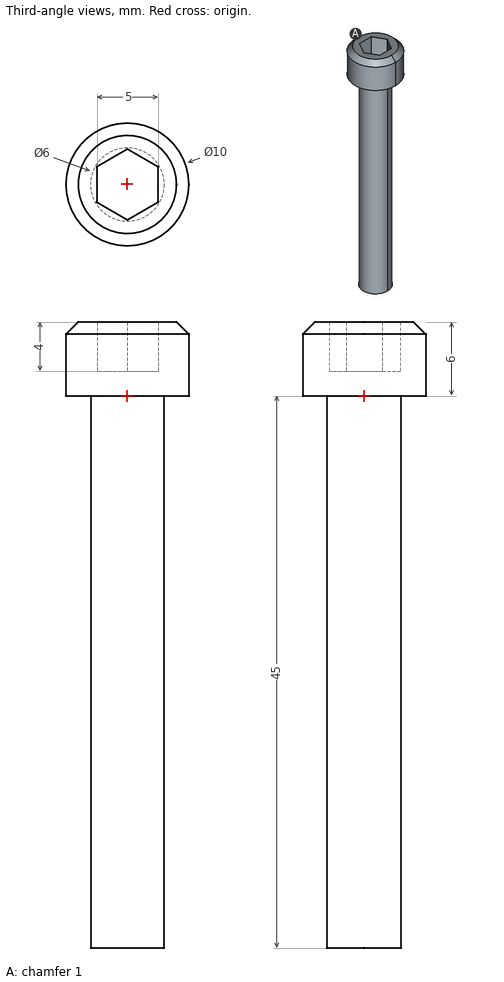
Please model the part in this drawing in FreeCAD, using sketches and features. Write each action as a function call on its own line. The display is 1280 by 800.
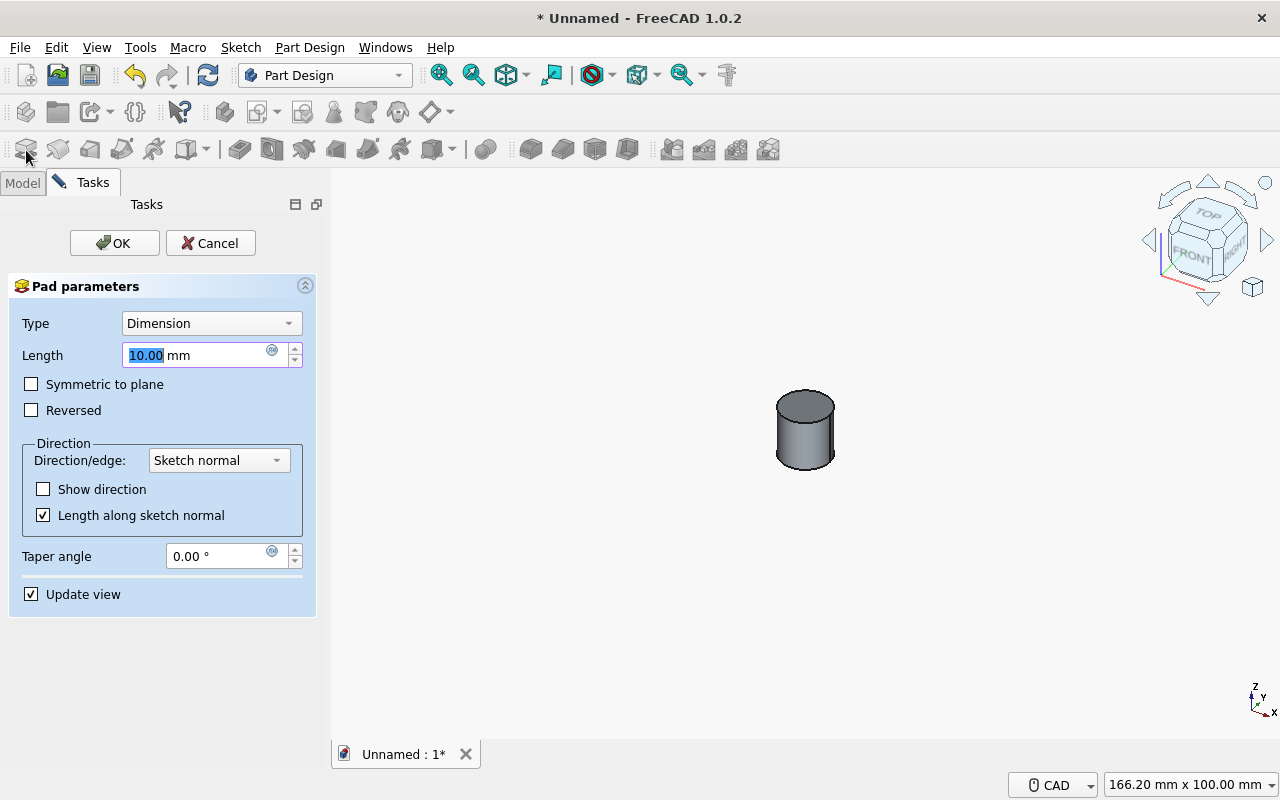
text(6)
key(Tab)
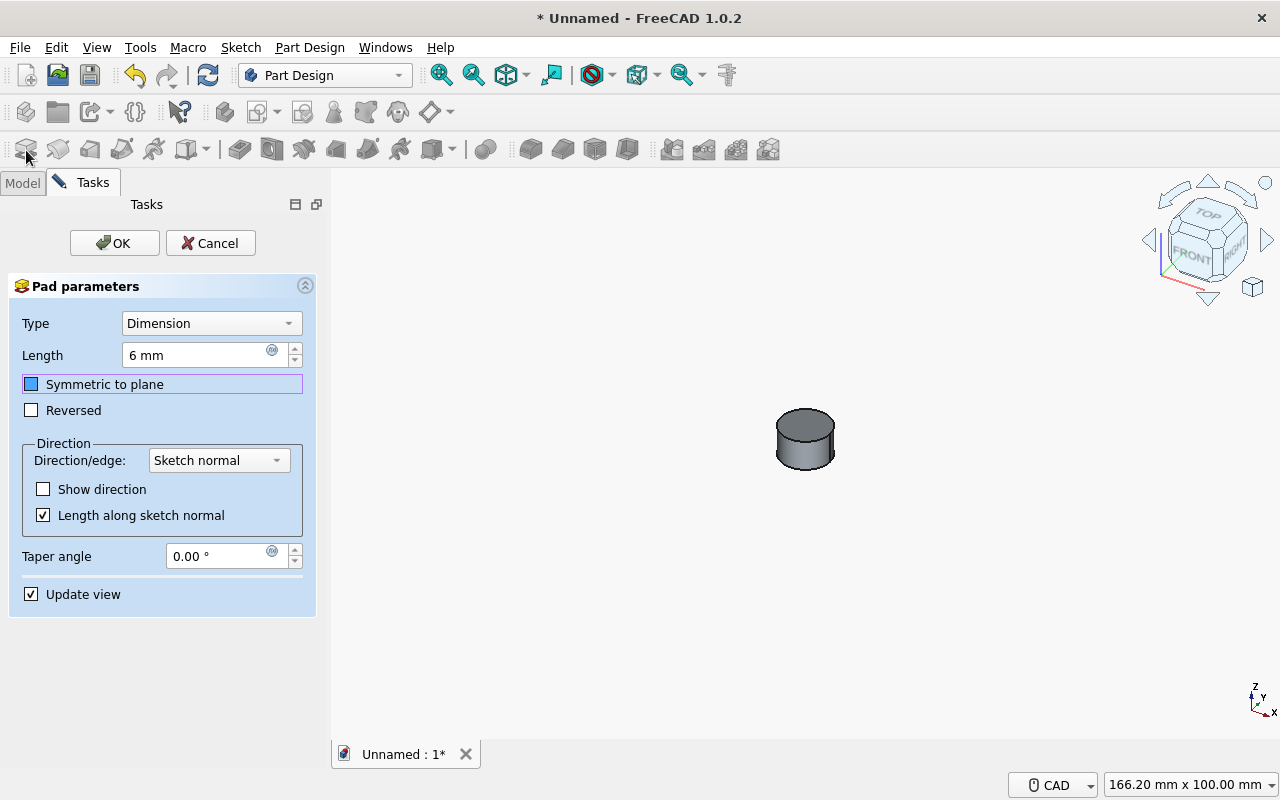
click(115, 243)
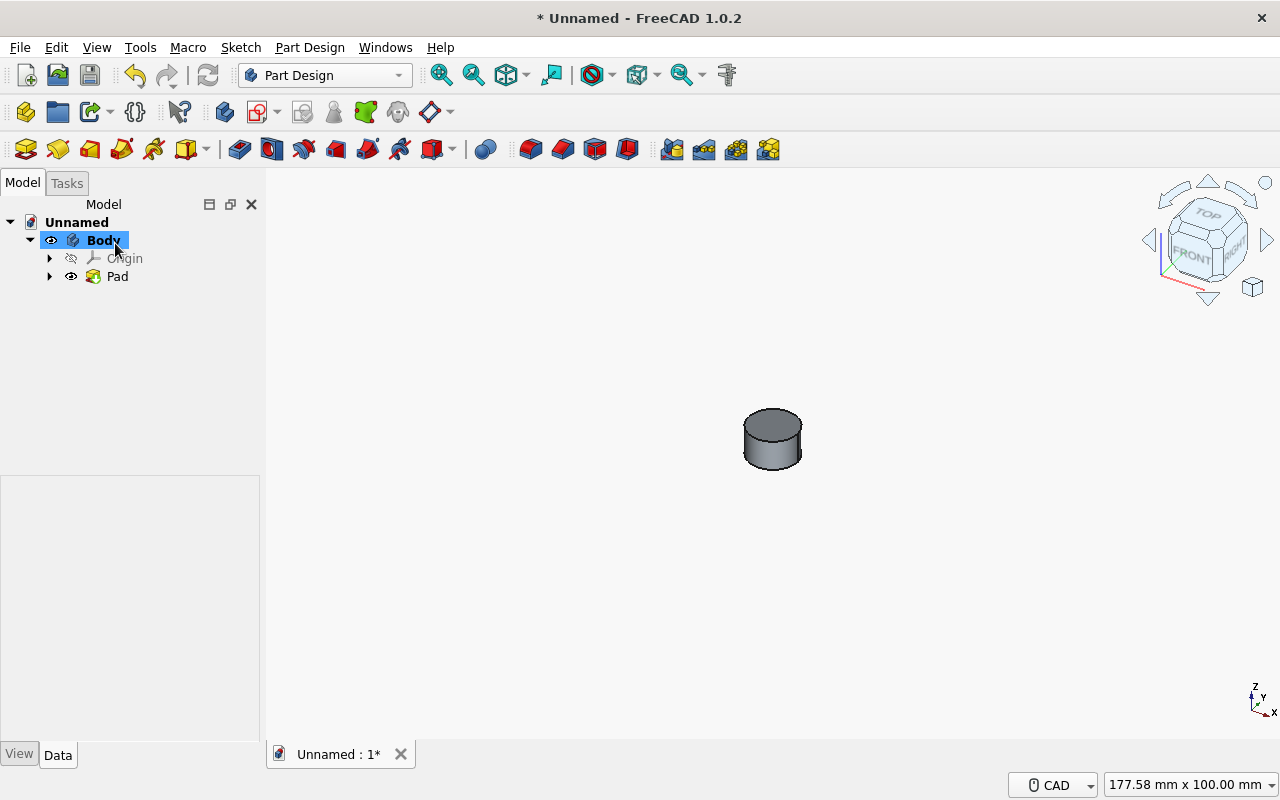
click(442, 76)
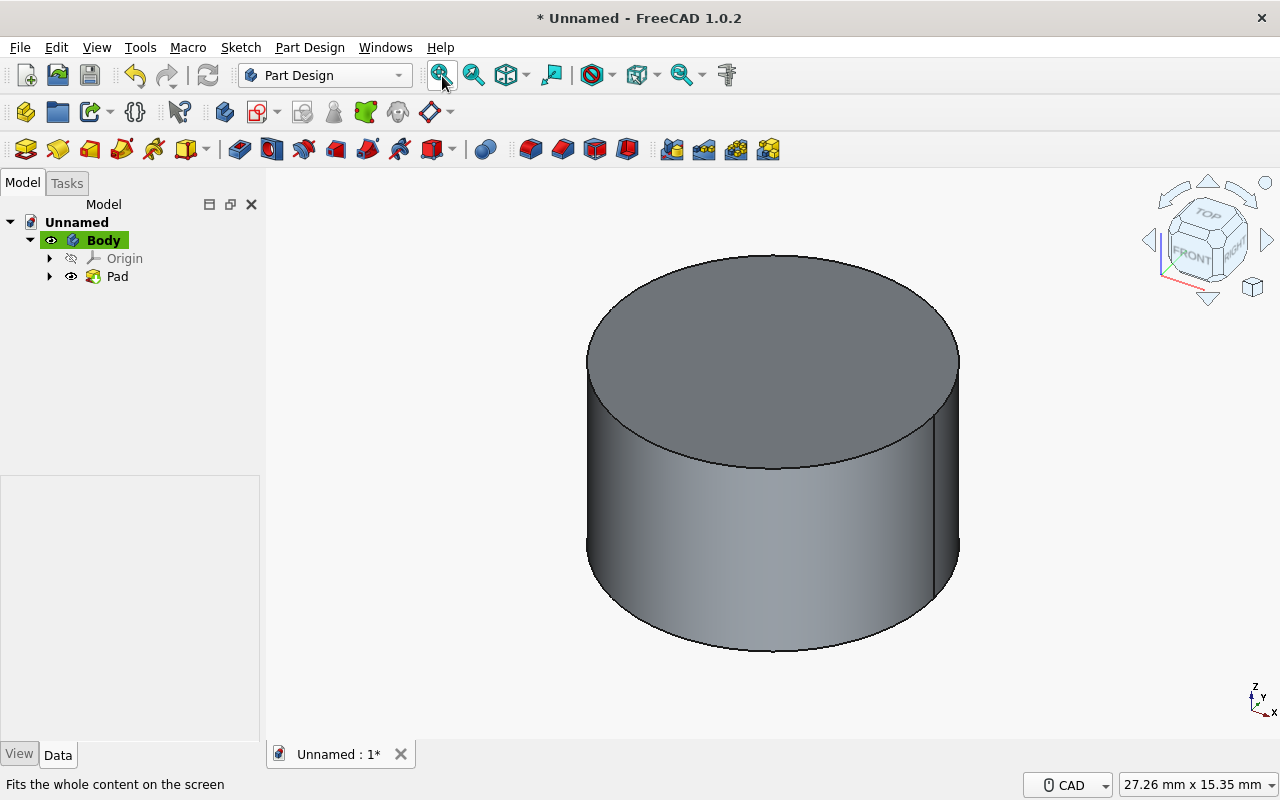
click(773, 361)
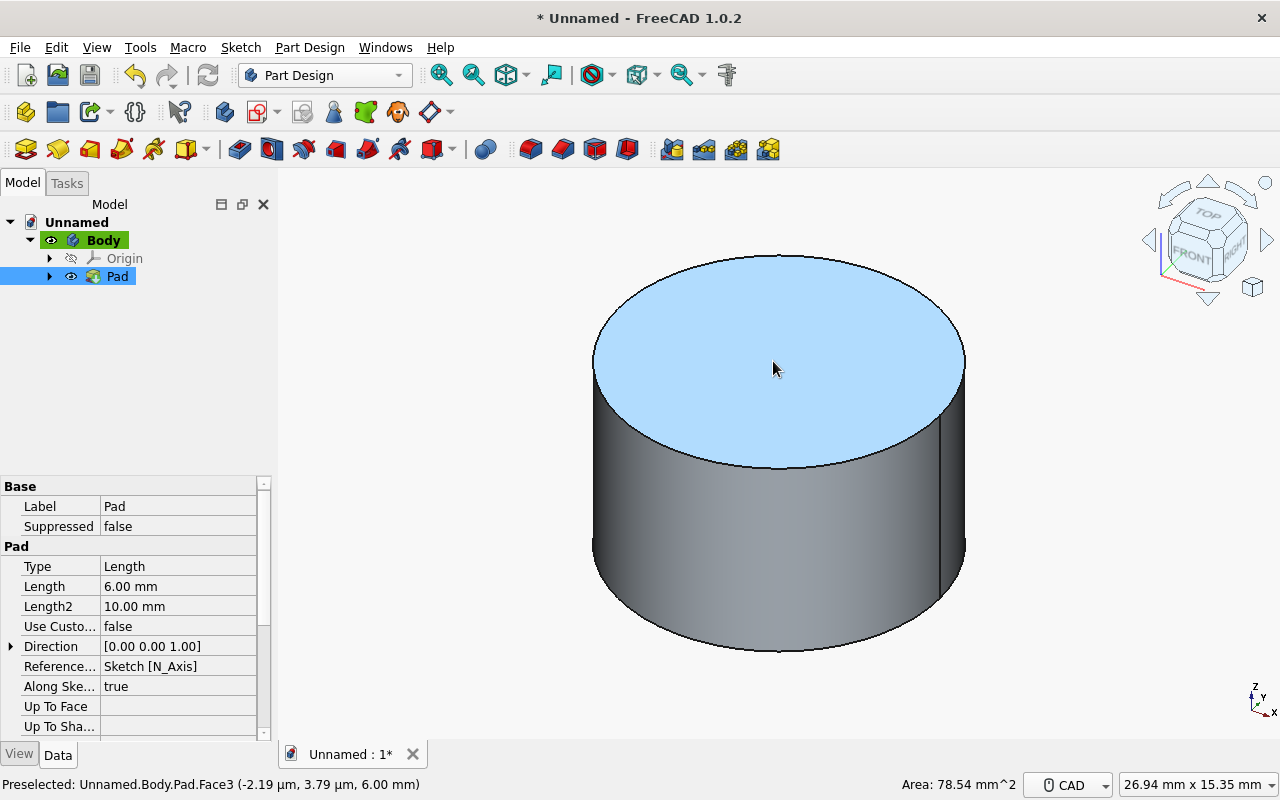
click(258, 112)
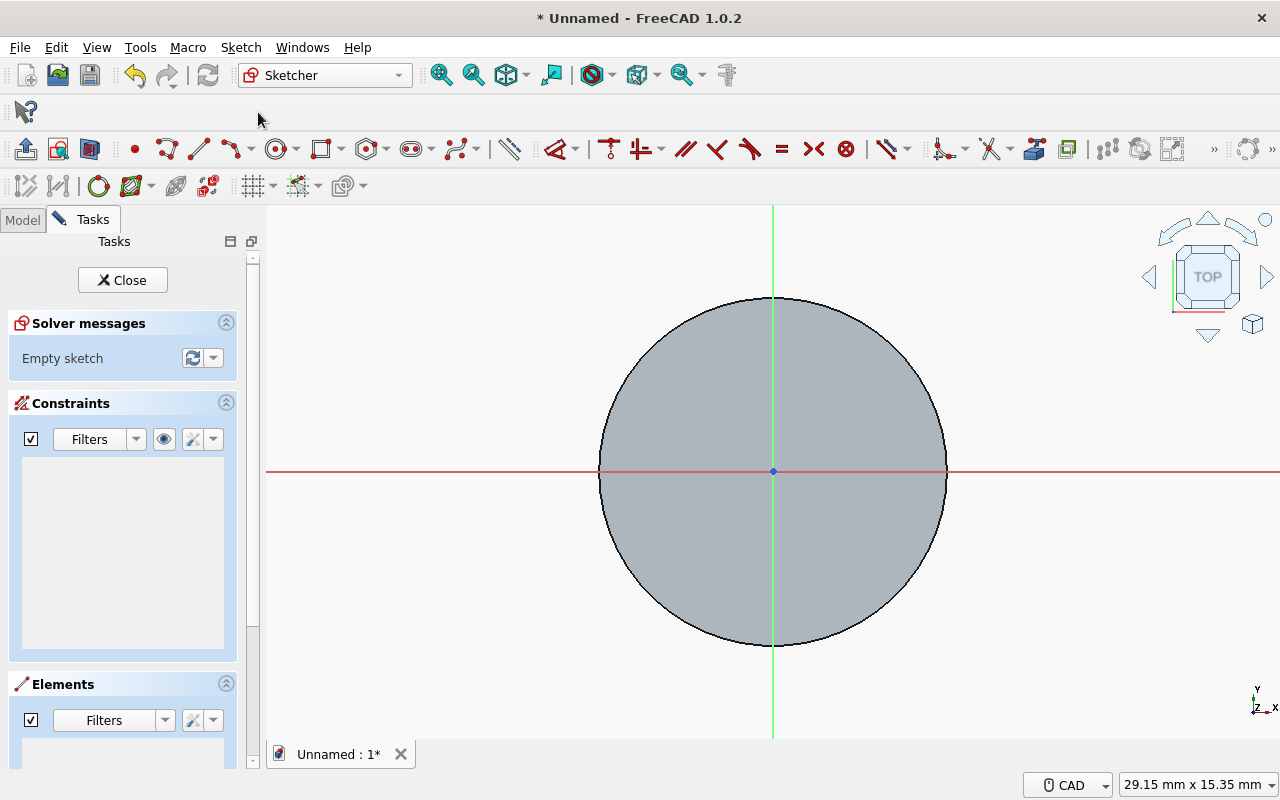
scroll(856, 472, up, 3)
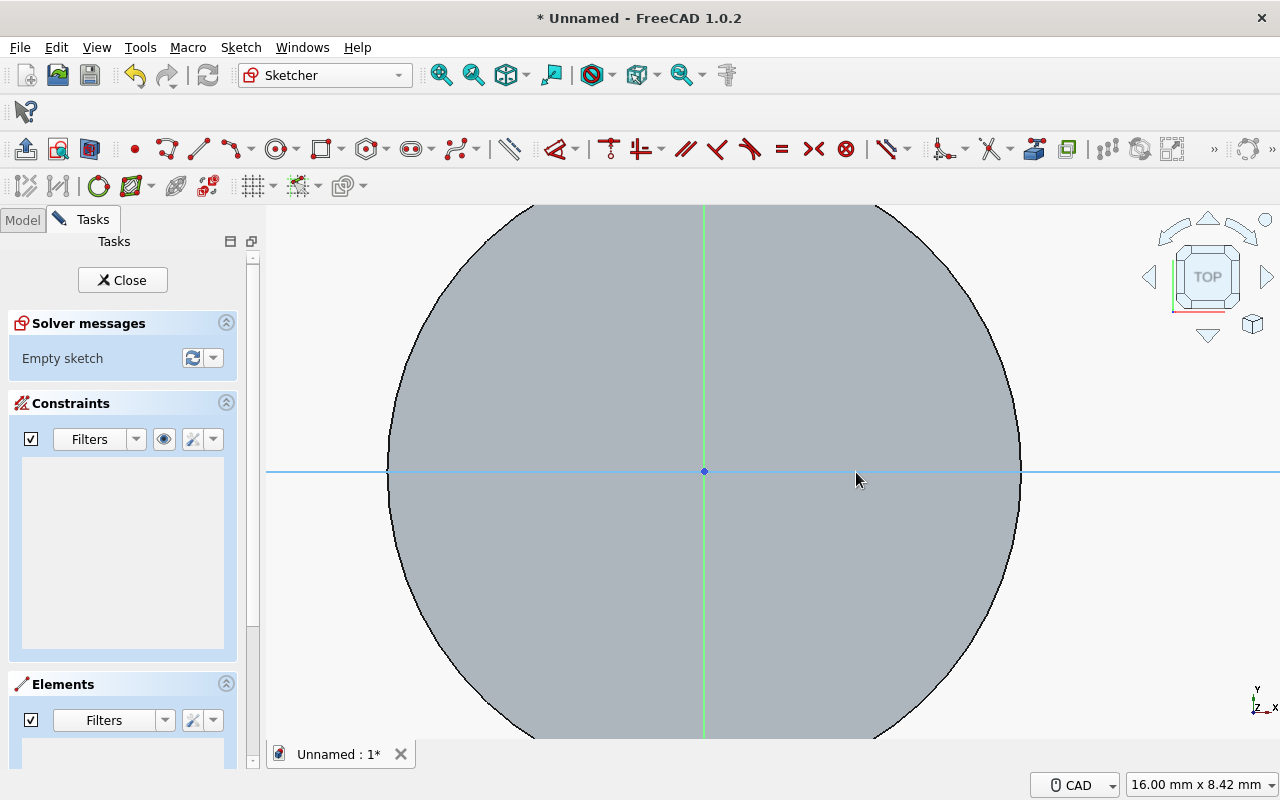
click(366, 150)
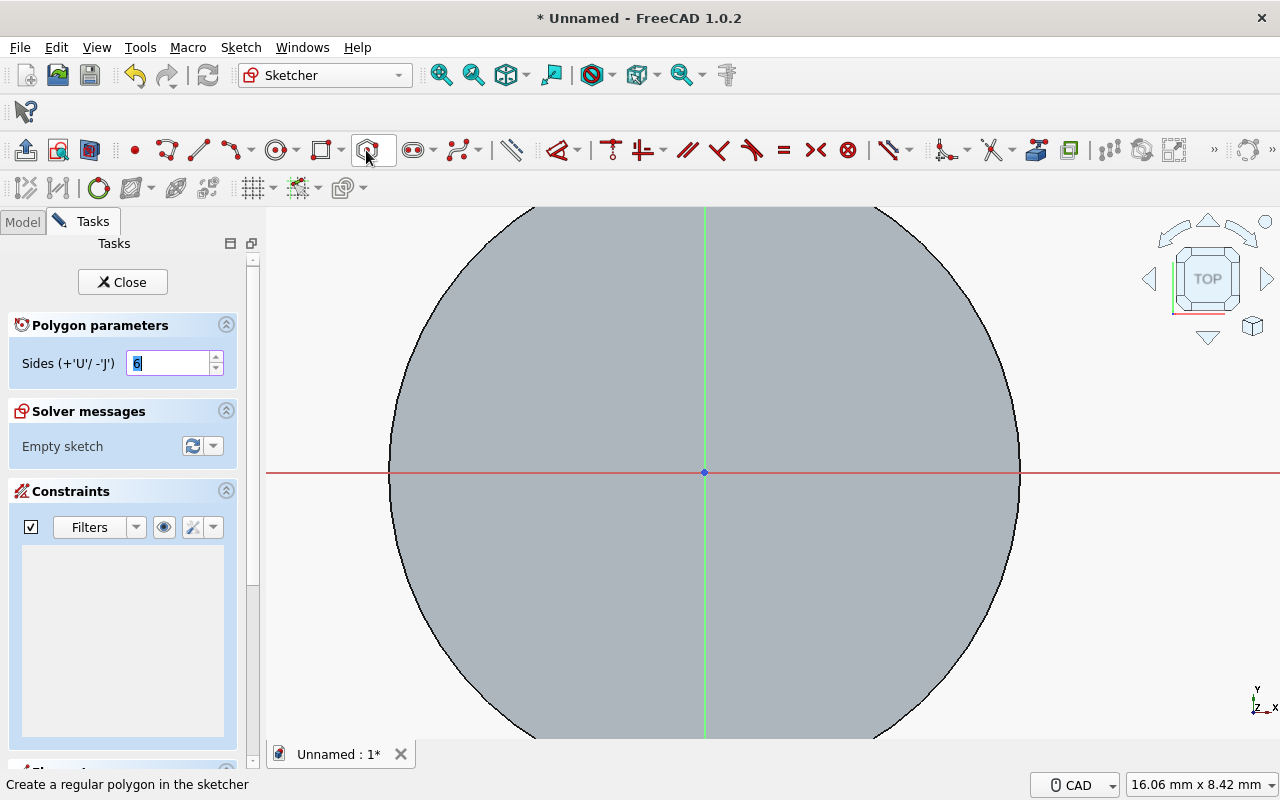
click(705, 473)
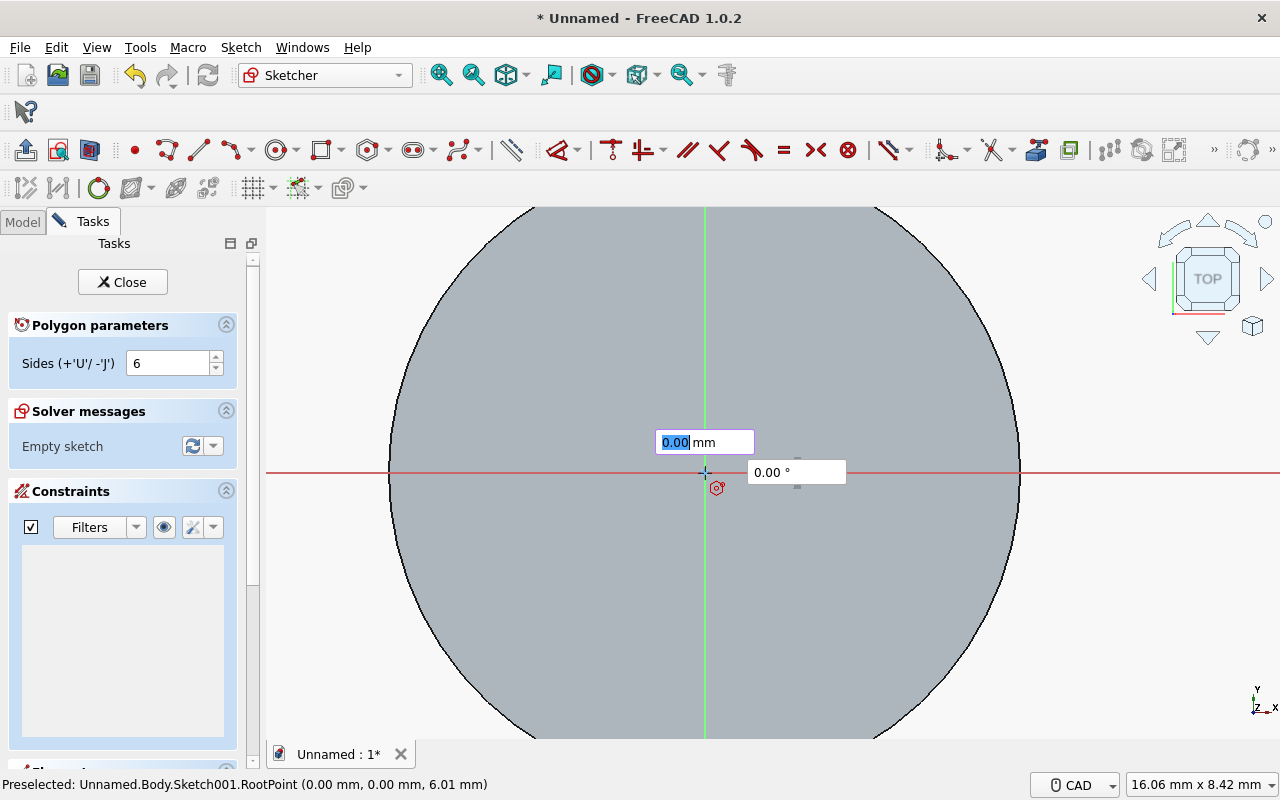
click(705, 290)
right_click(705, 290)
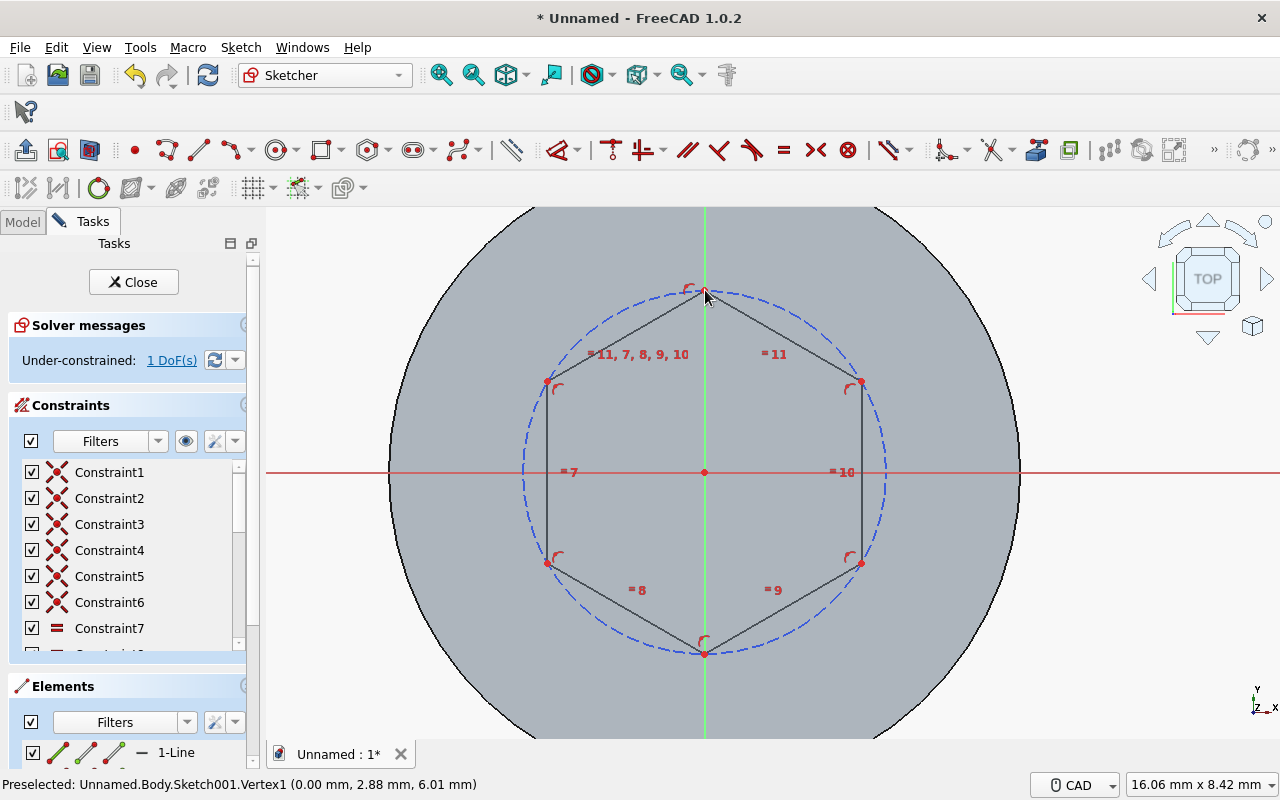
click(547, 382)